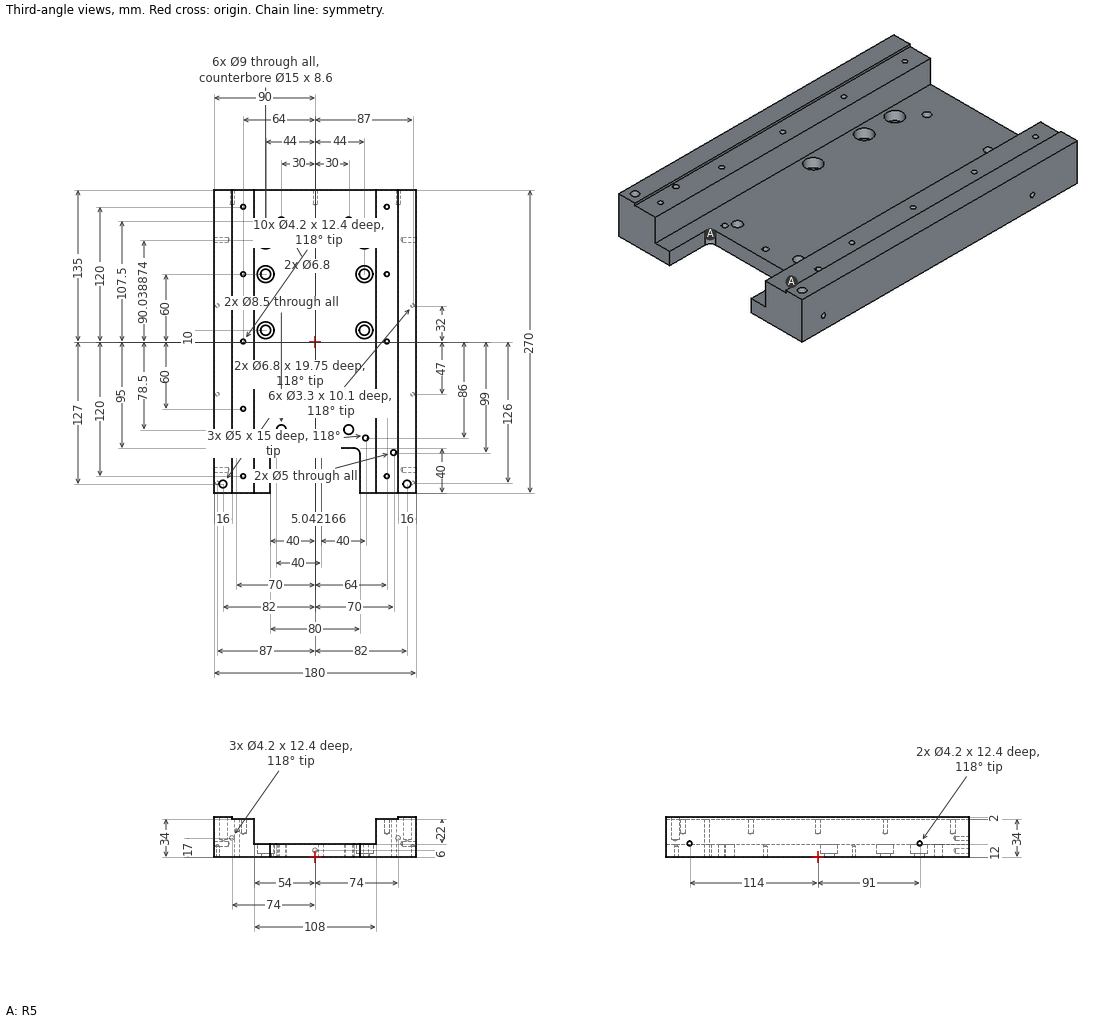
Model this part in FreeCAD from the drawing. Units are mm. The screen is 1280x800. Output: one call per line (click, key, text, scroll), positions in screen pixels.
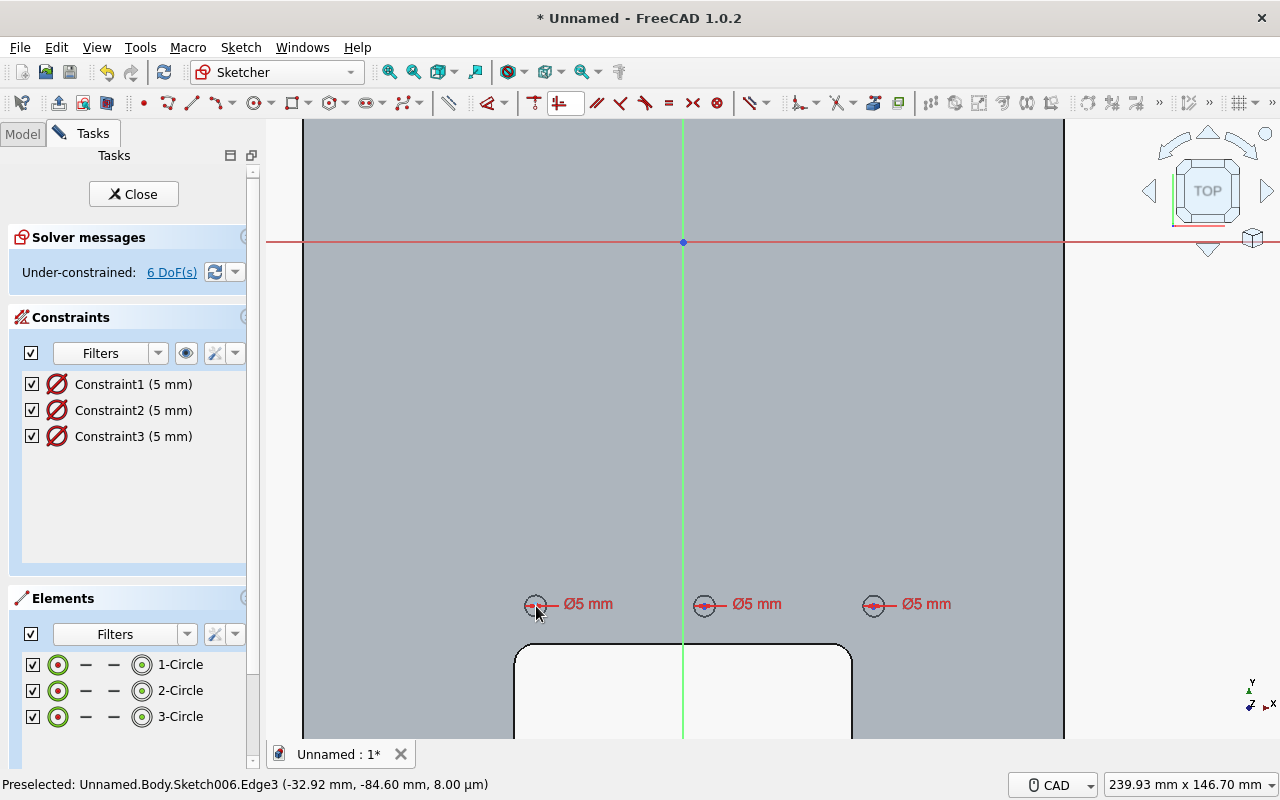
click(874, 606)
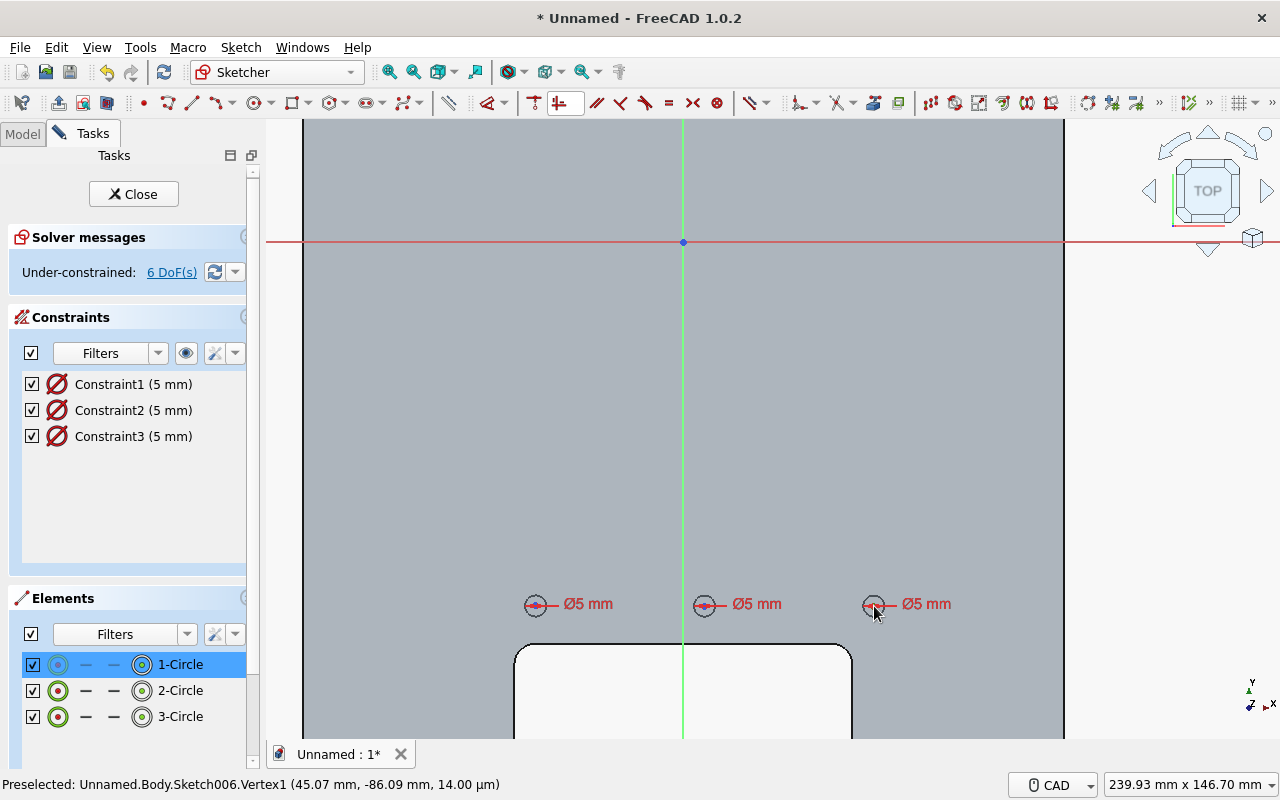
click(704, 606)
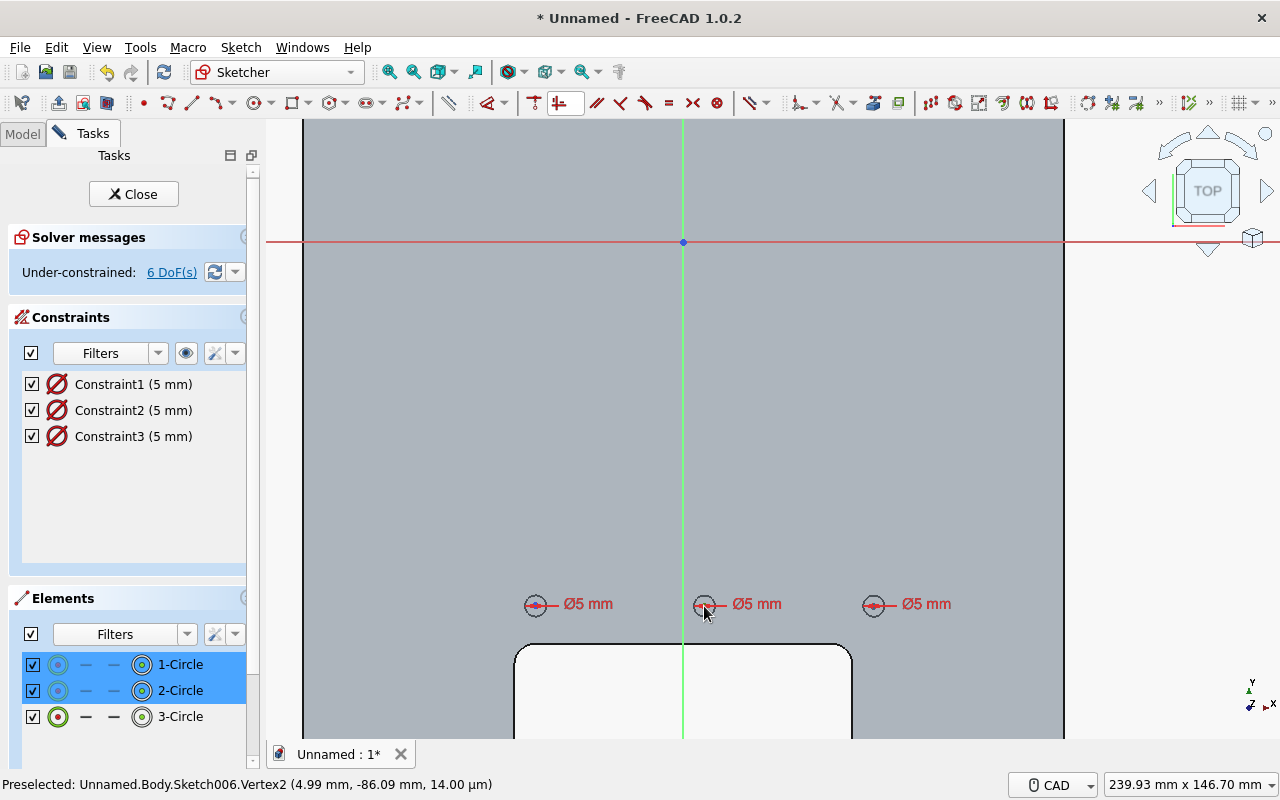
key(h)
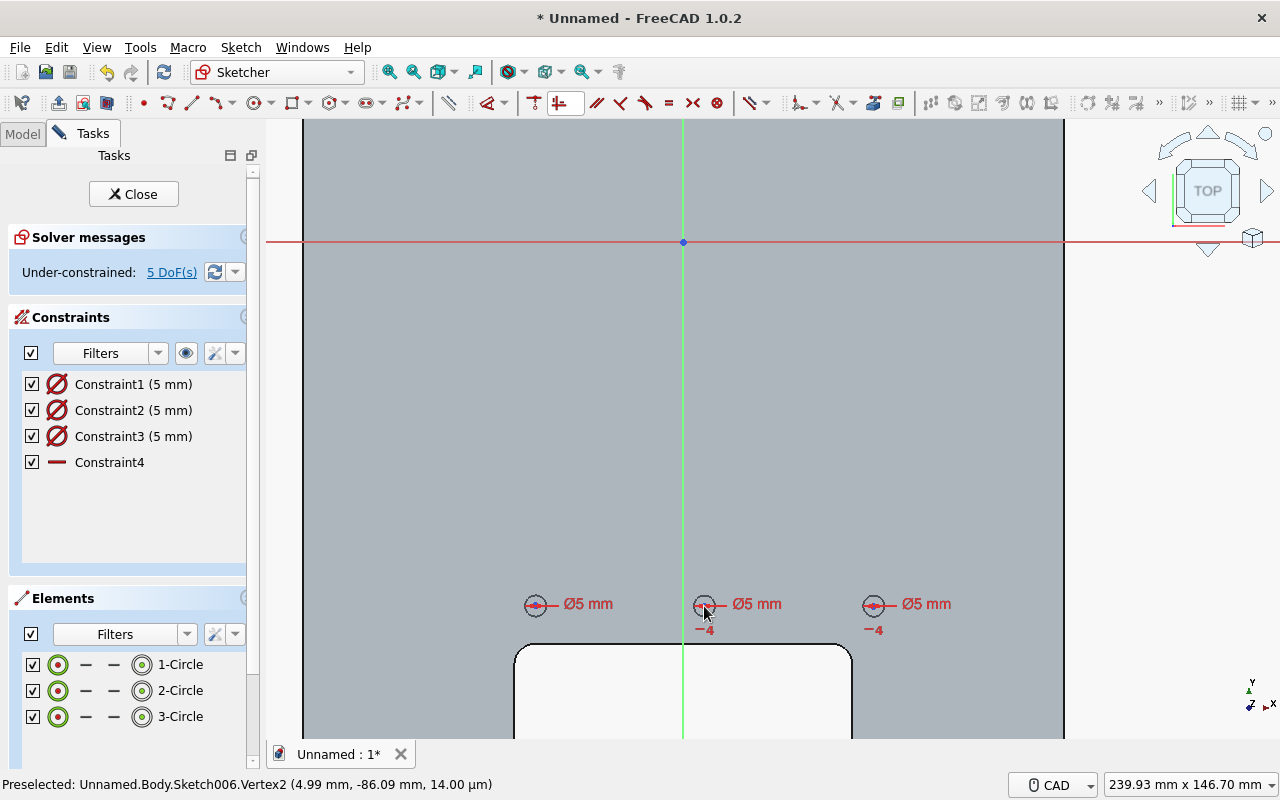
click(704, 606)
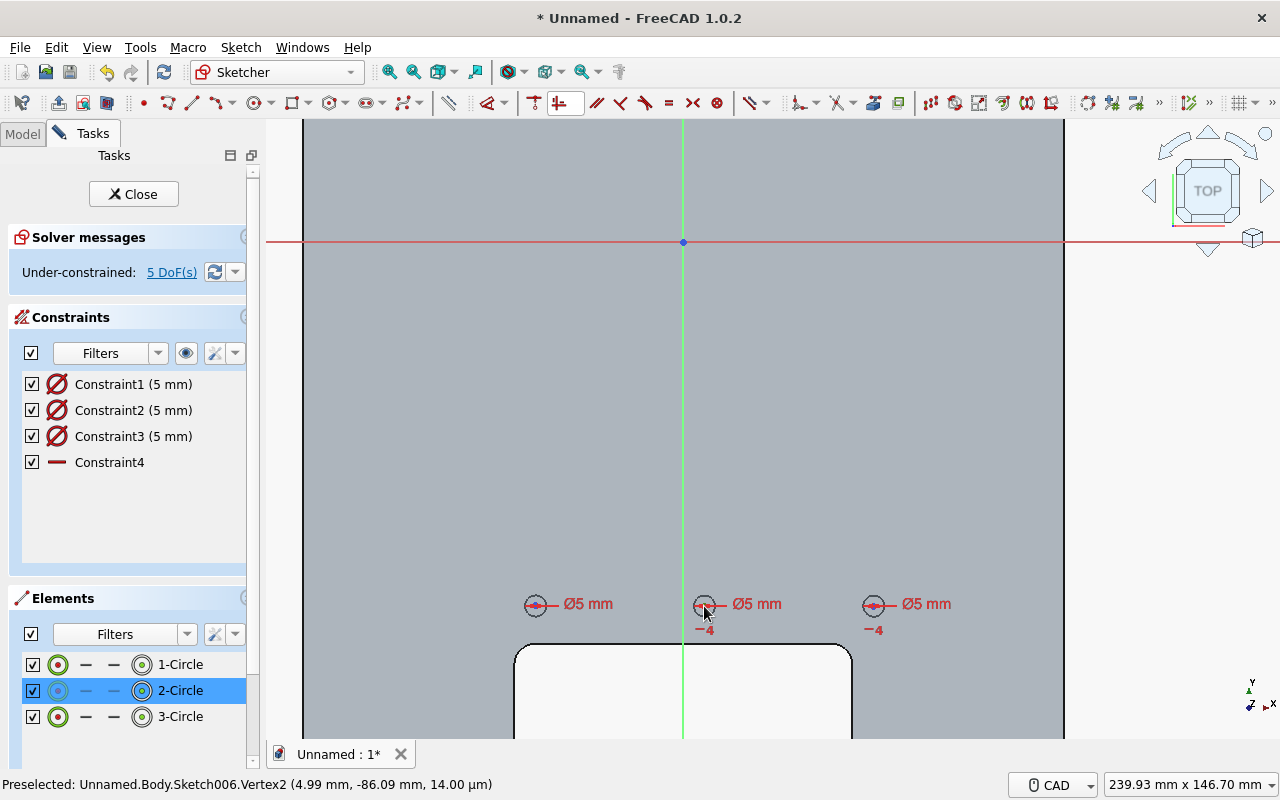
click(536, 606)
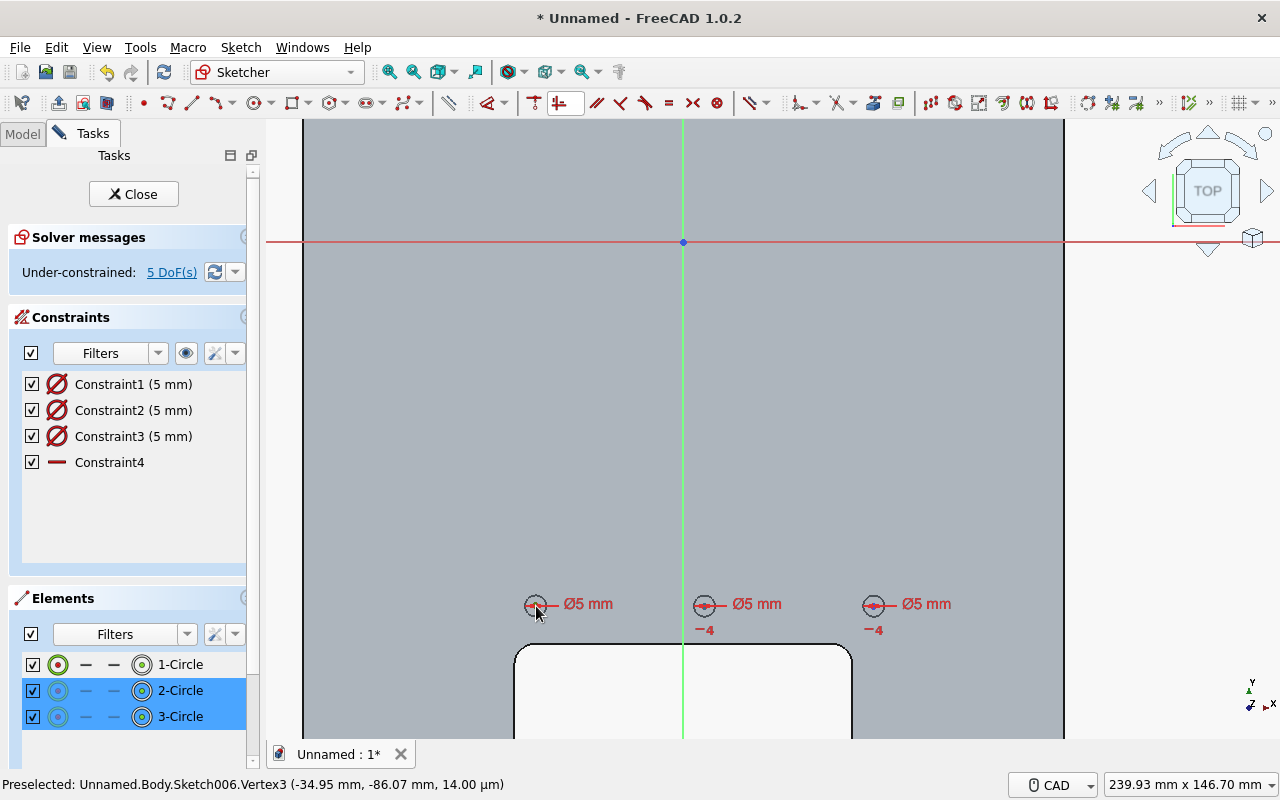
click(578, 104)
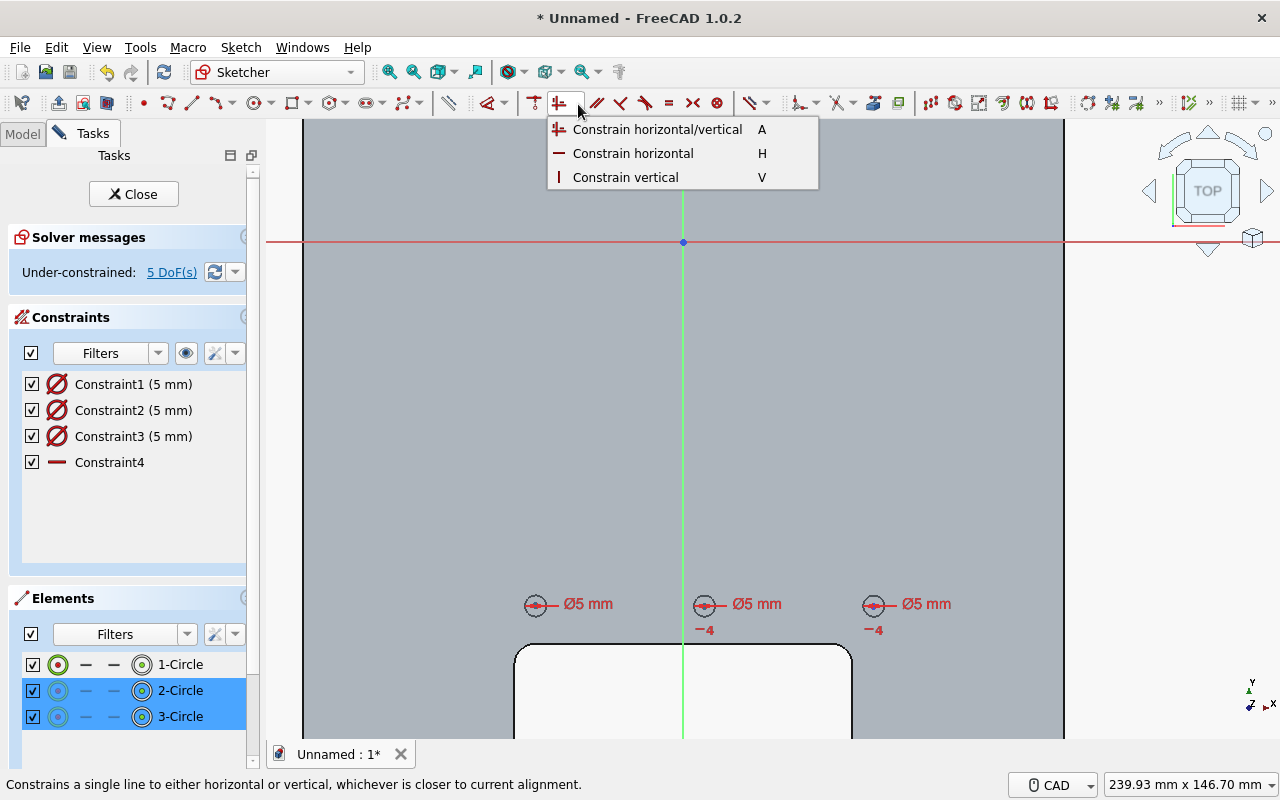
click(683, 153)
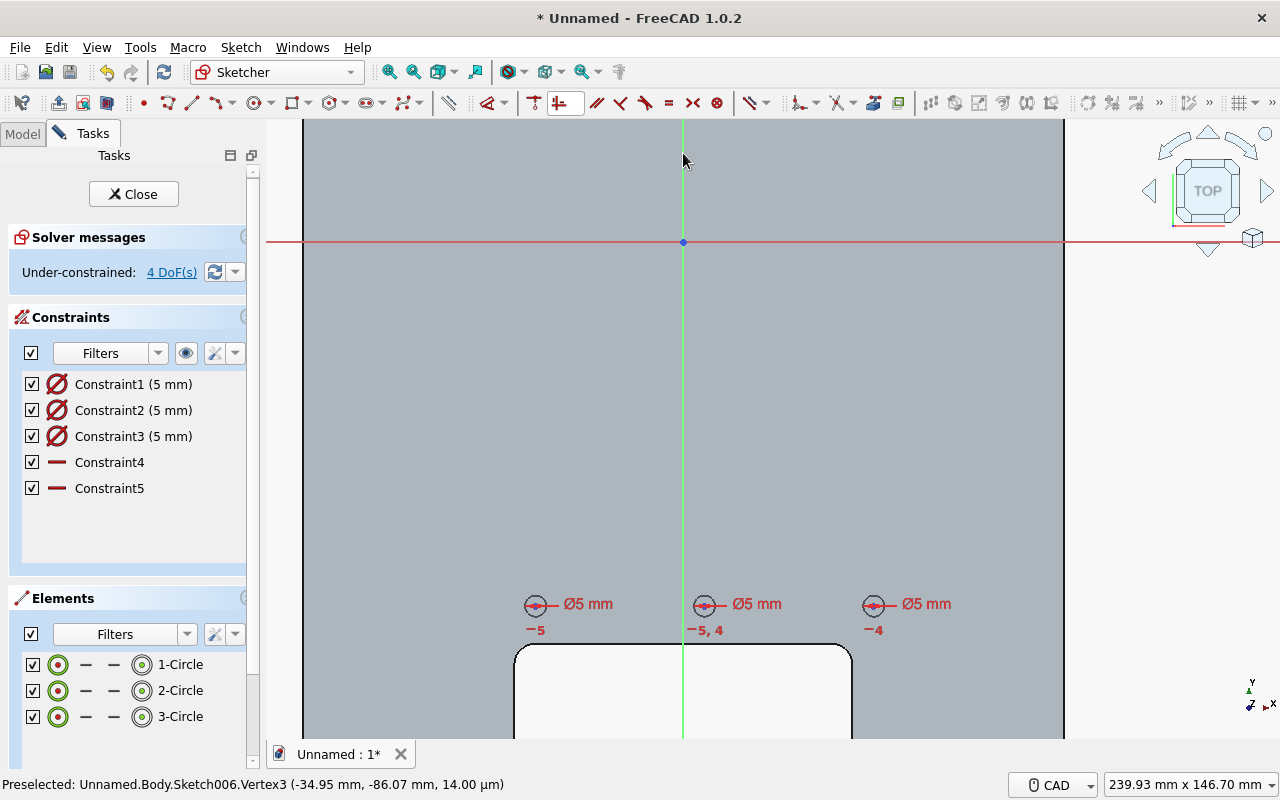
click(488, 104)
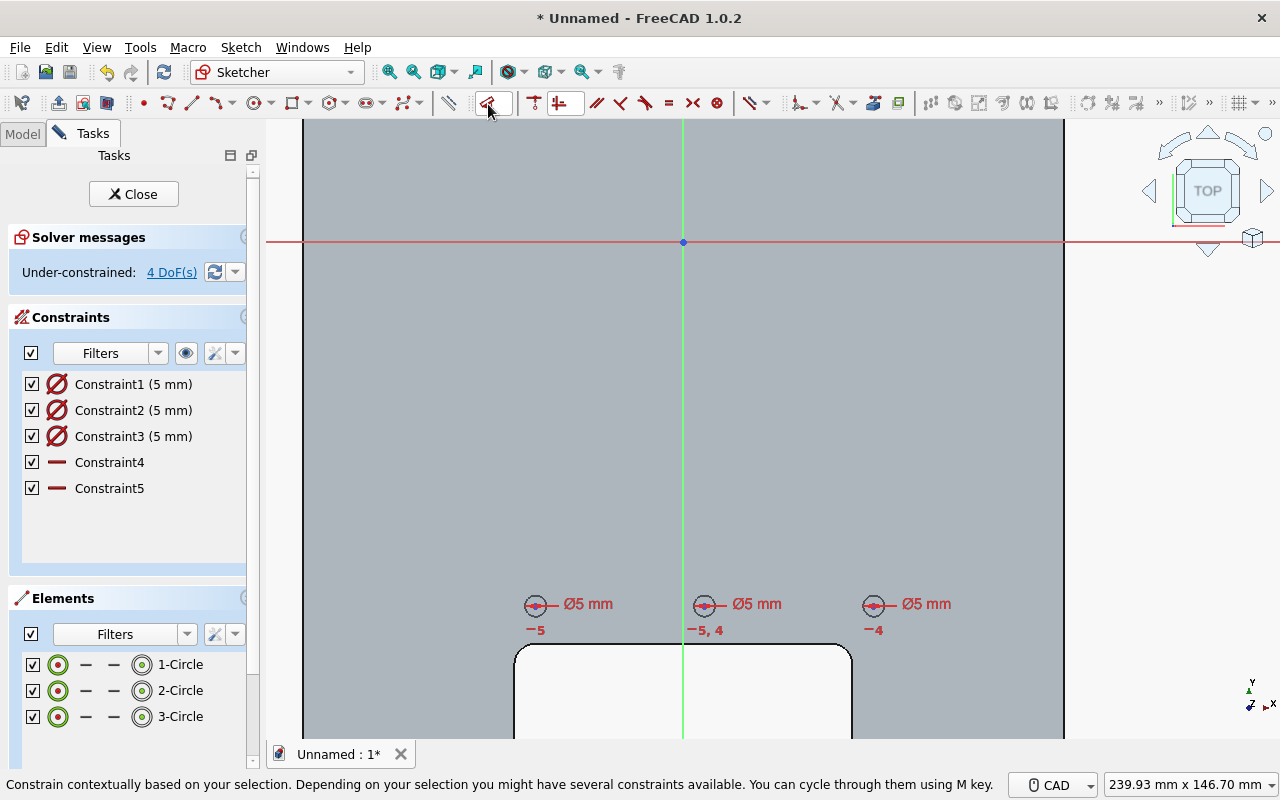
click(874, 606)
click(908, 424)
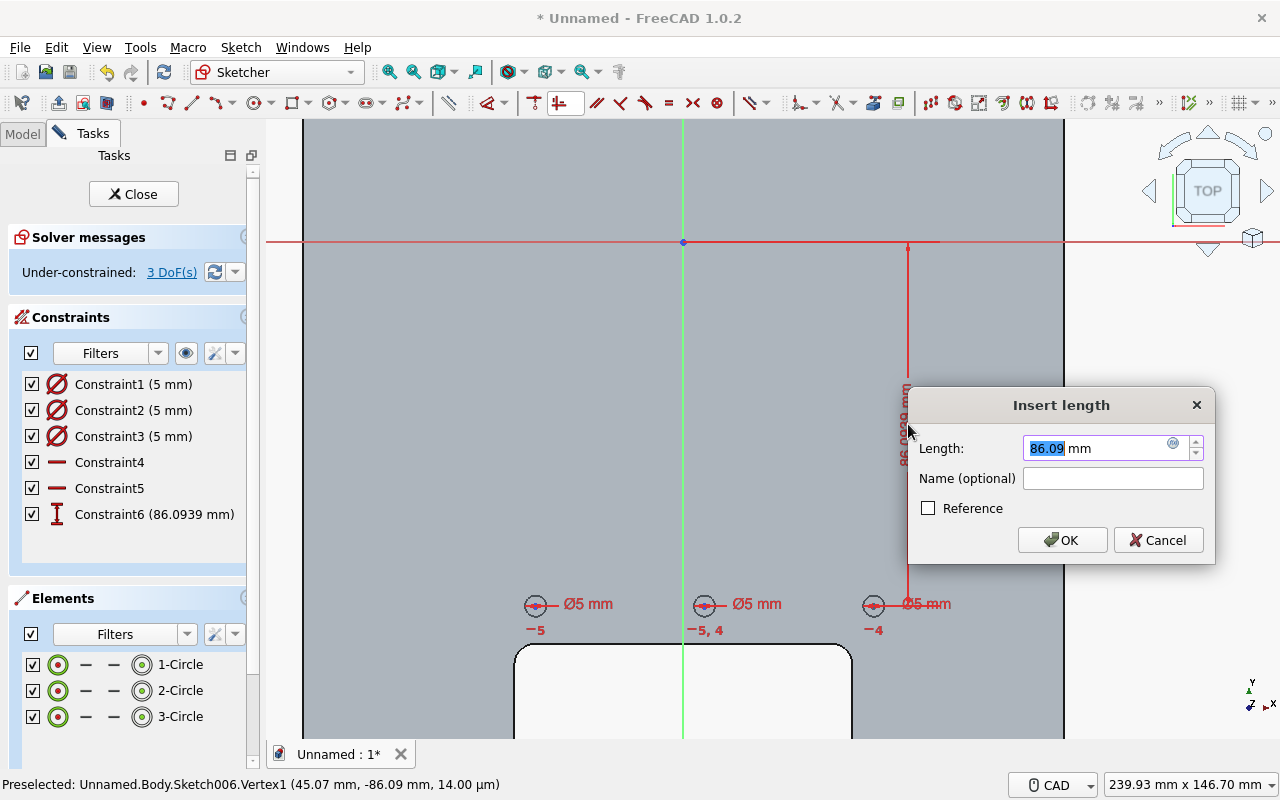
text(86)
key(Return)